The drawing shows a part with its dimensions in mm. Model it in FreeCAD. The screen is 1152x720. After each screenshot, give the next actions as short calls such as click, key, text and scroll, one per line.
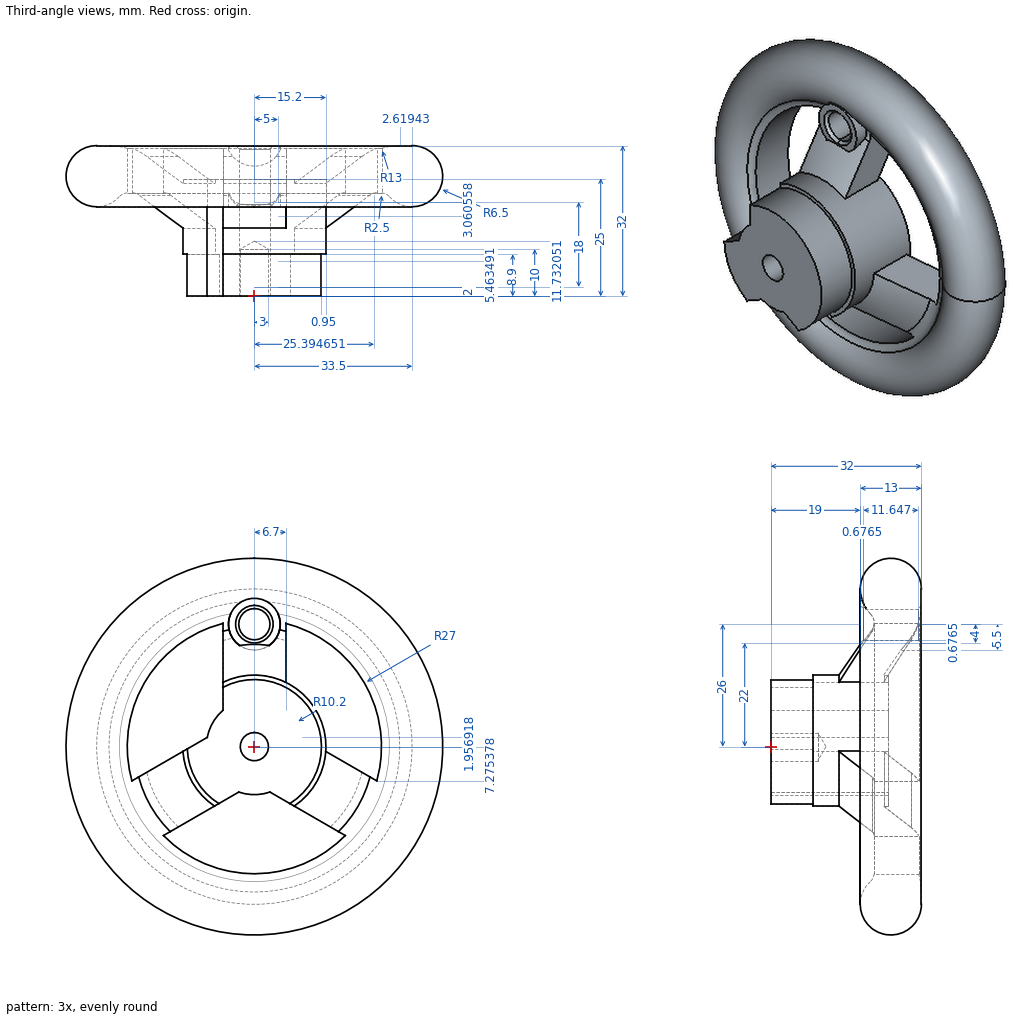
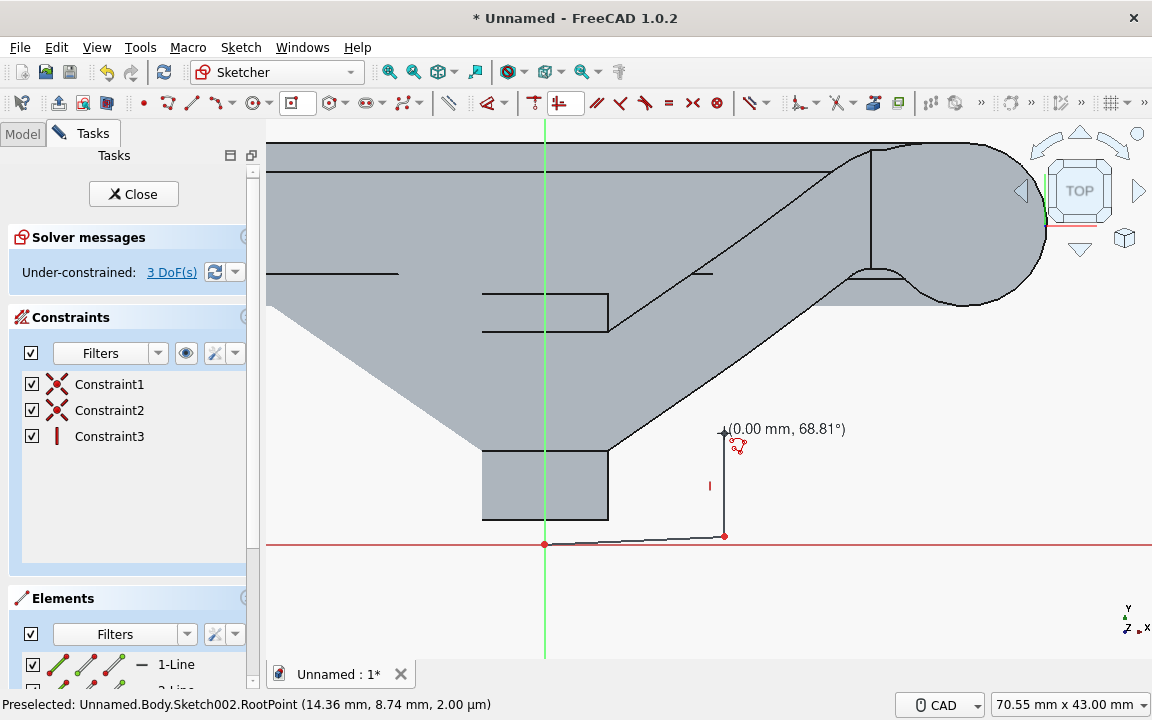
scroll(736, 433, up, 2)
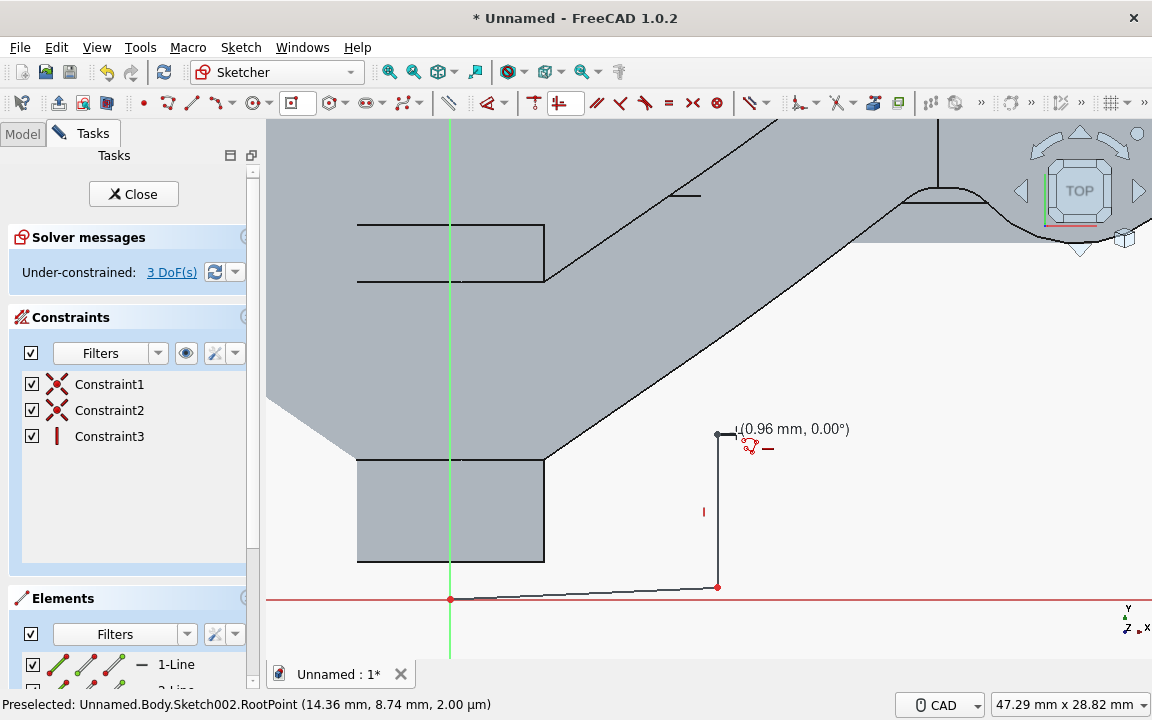
click(735, 433)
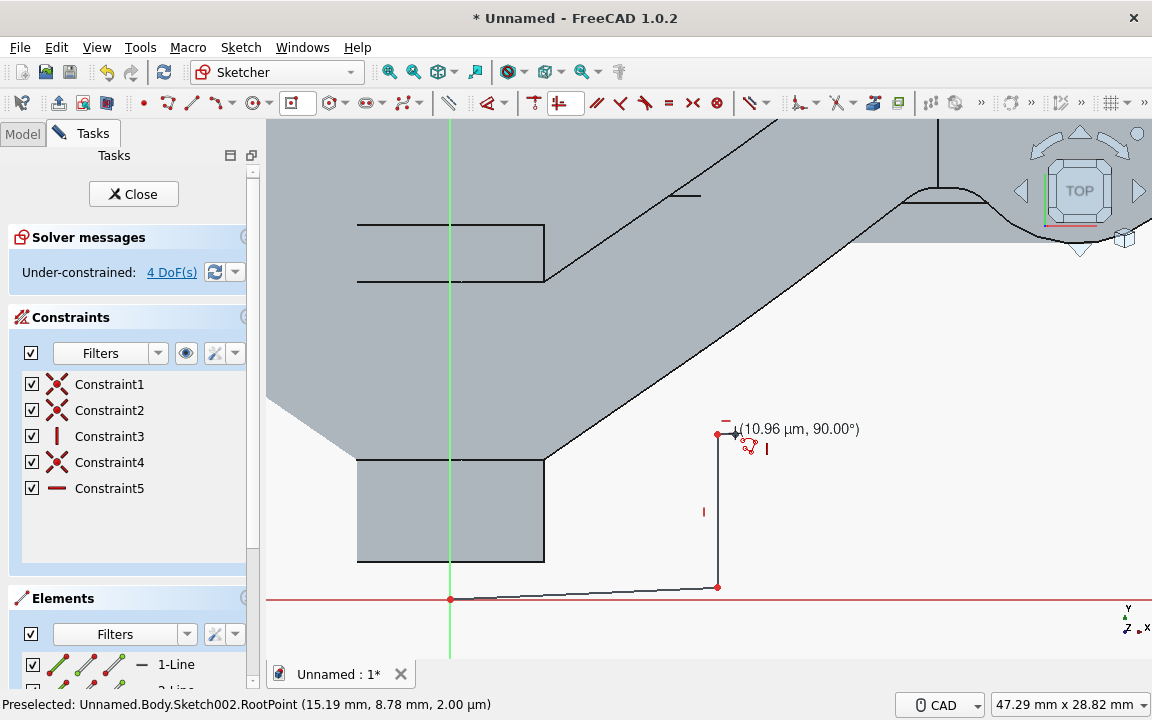
scroll(738, 437, down, 2)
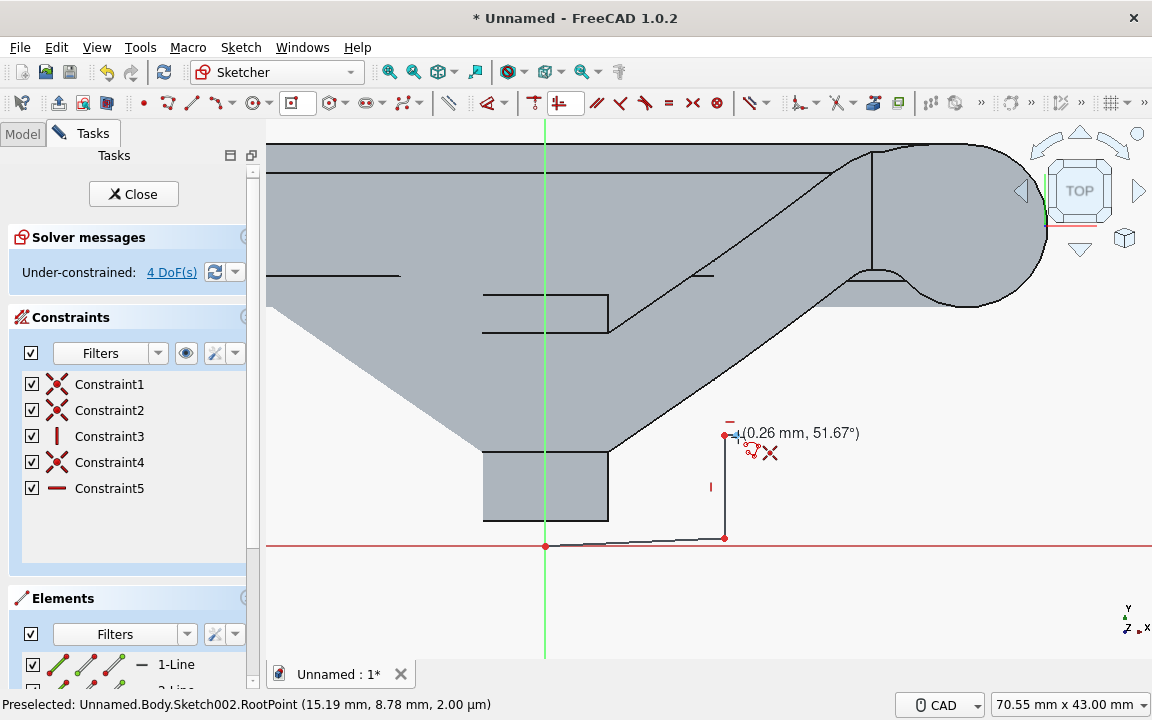
click(736, 232)
click(554, 232)
click(545, 546)
key(Escape)
key(Escape)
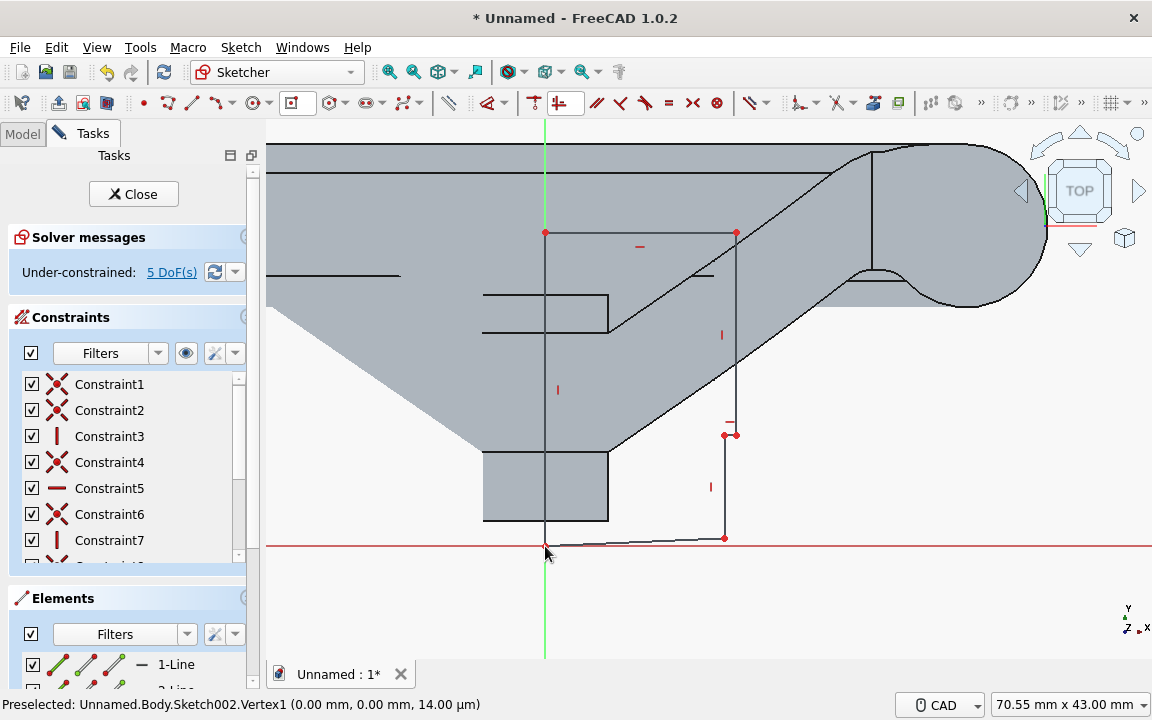
click(599, 544)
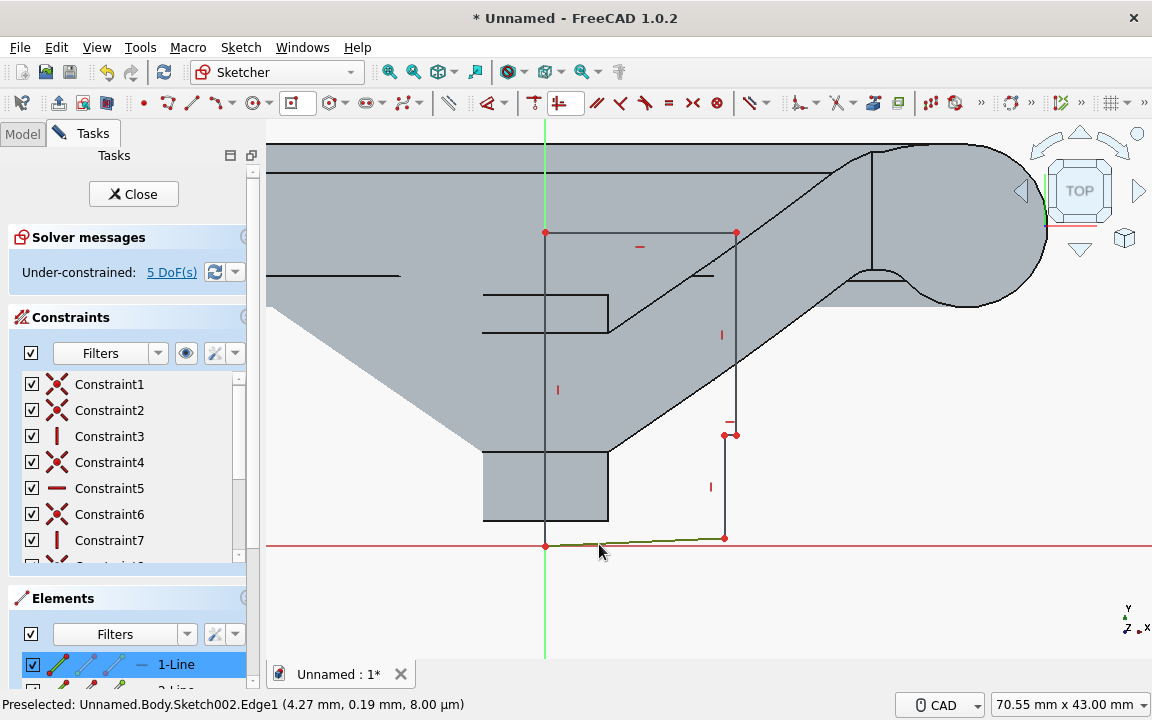
key(h)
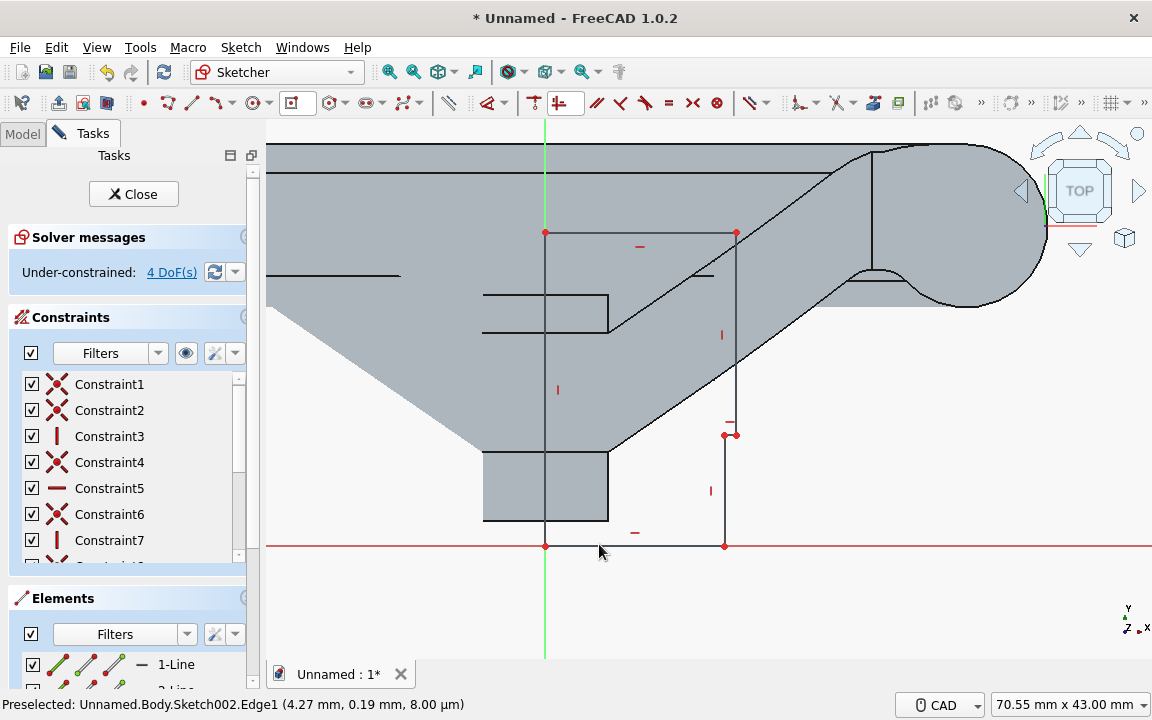
key(d)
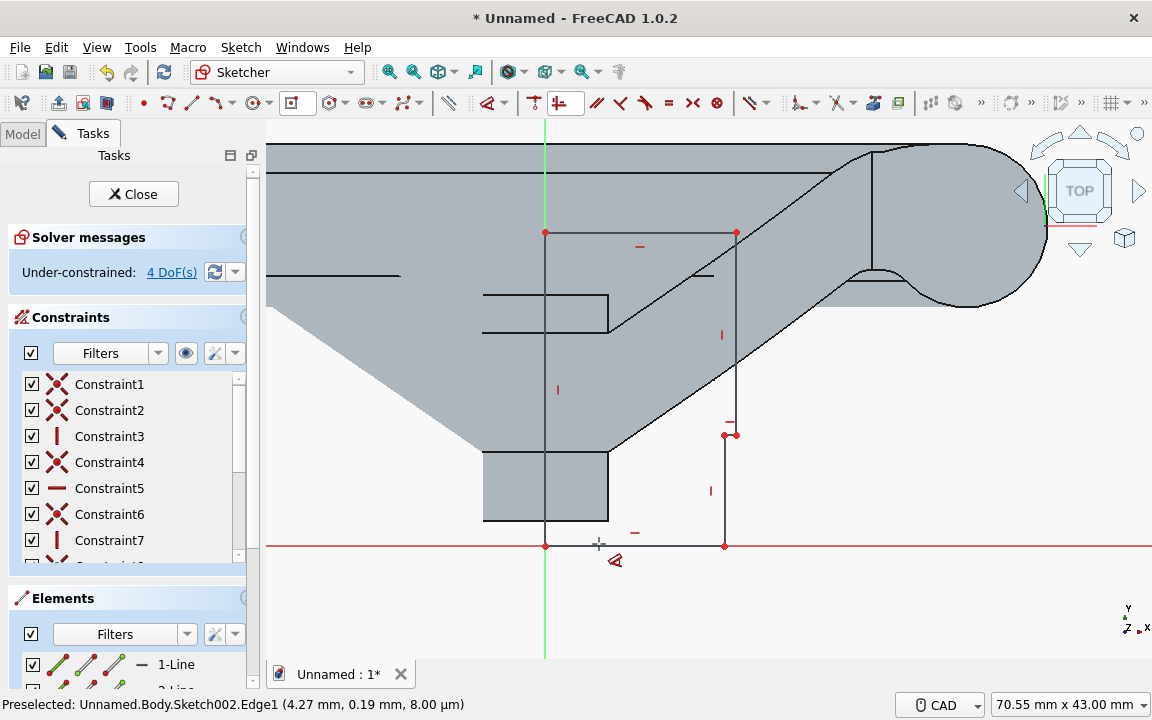
click(545, 327)
click(511, 390)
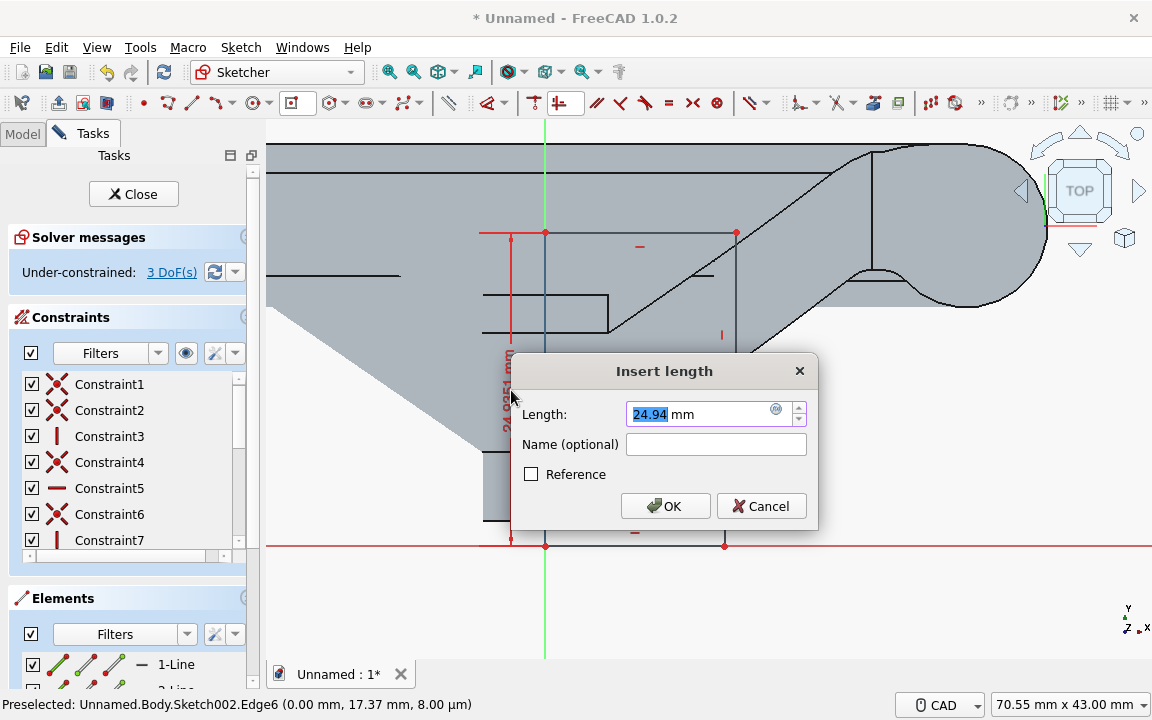
text(25)
key(Return)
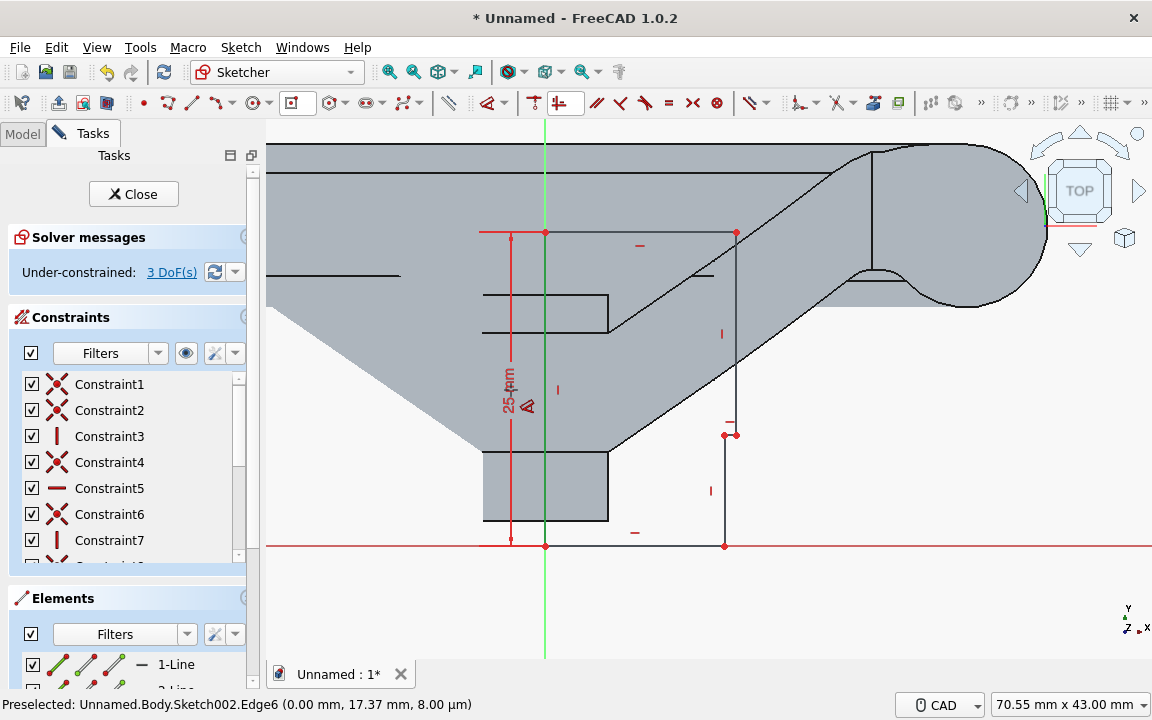
click(725, 513)
click(759, 491)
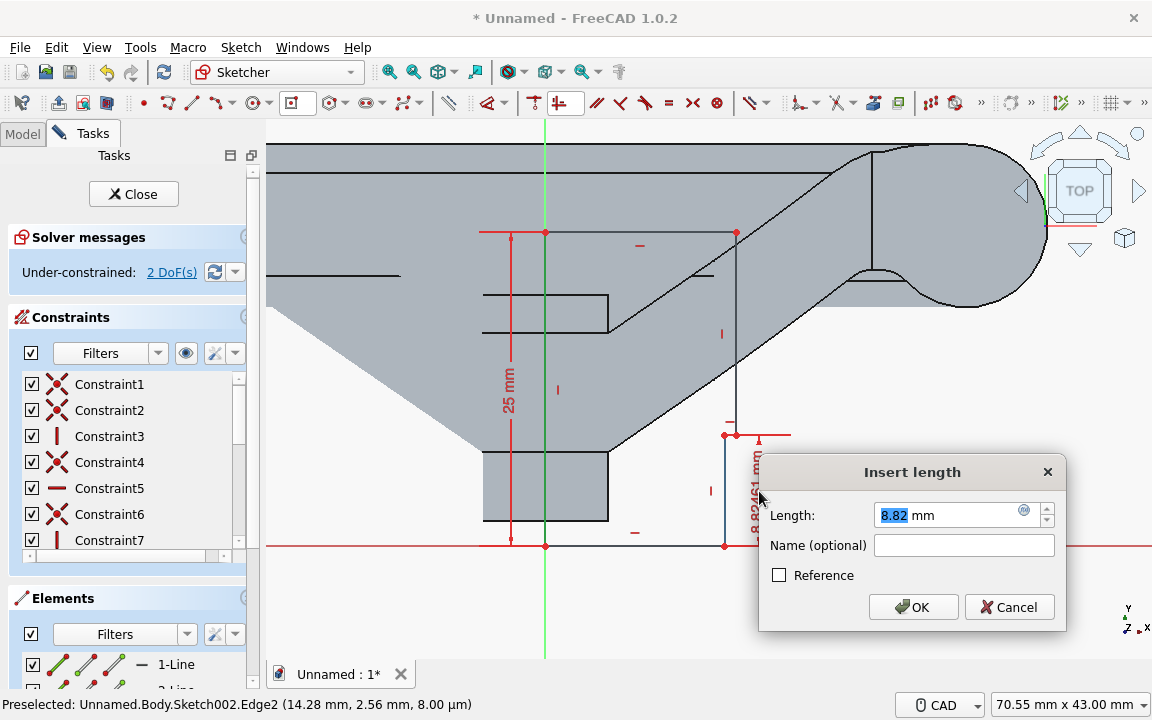
text(8.9)
key(Return)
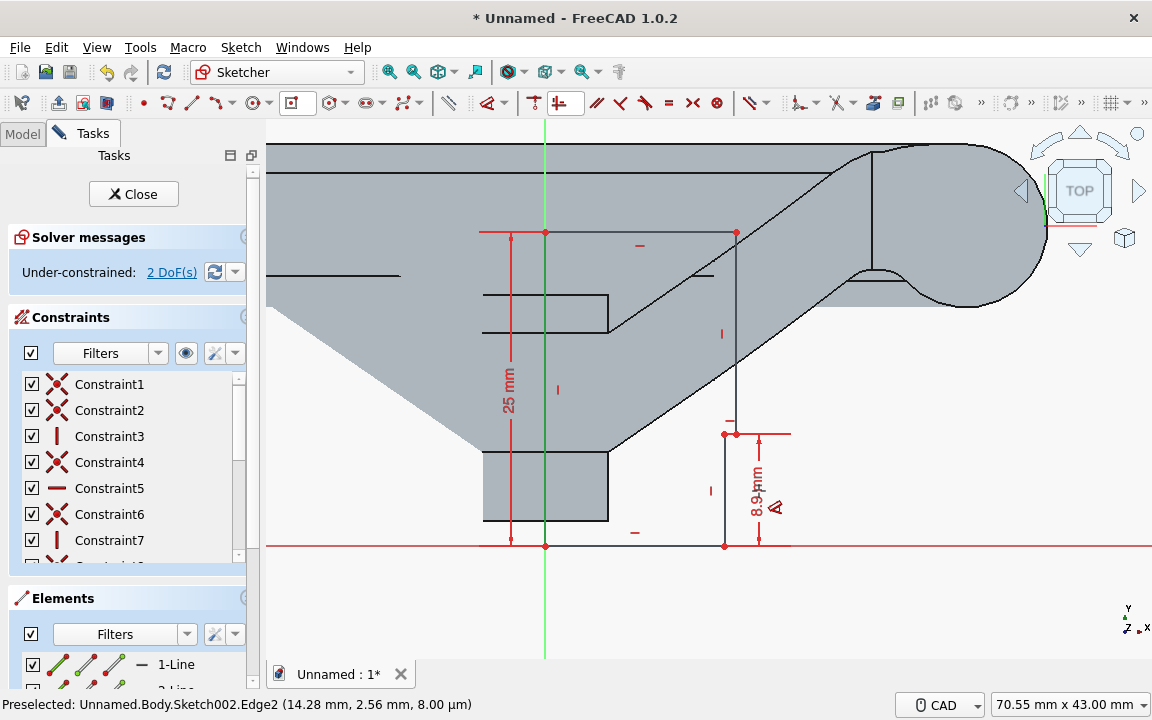
scroll(730, 434, up, 7)